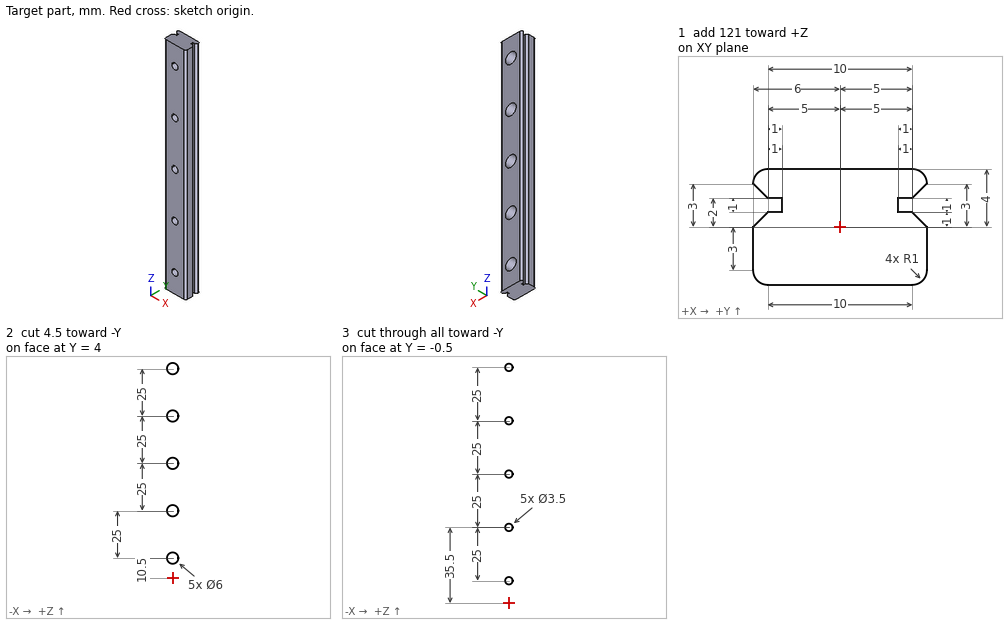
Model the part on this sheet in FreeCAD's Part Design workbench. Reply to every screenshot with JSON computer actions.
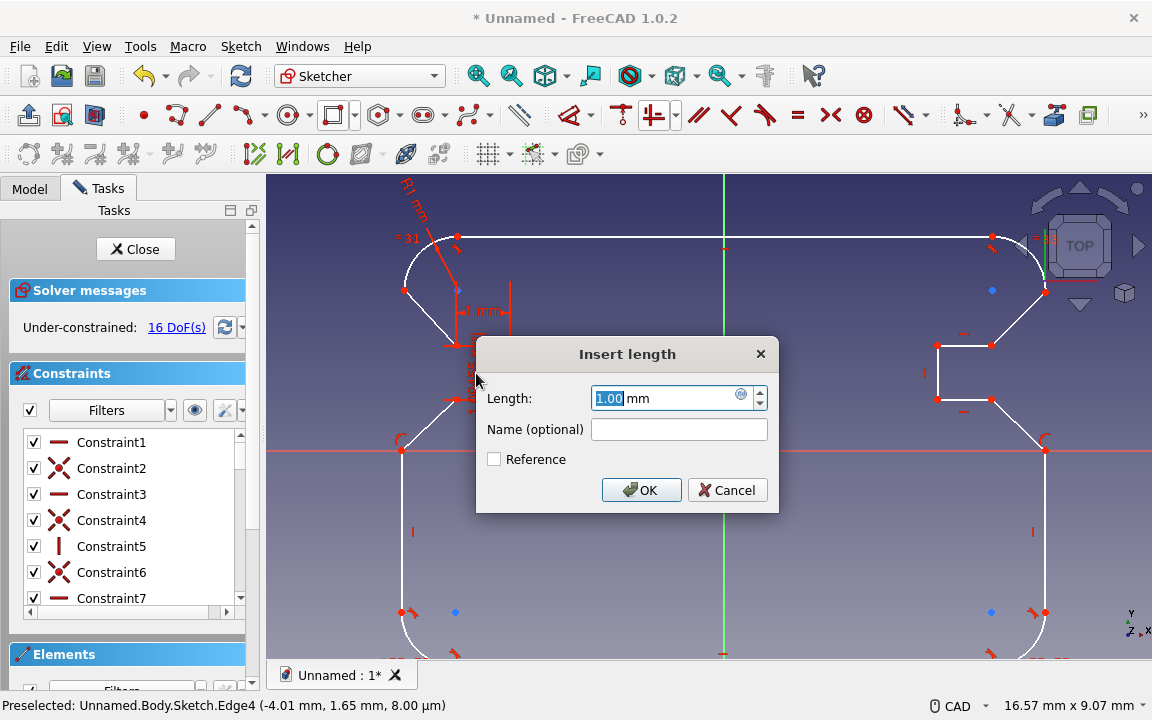
{"action": "type", "text": "1"}
{"action": "key", "text": "Return"}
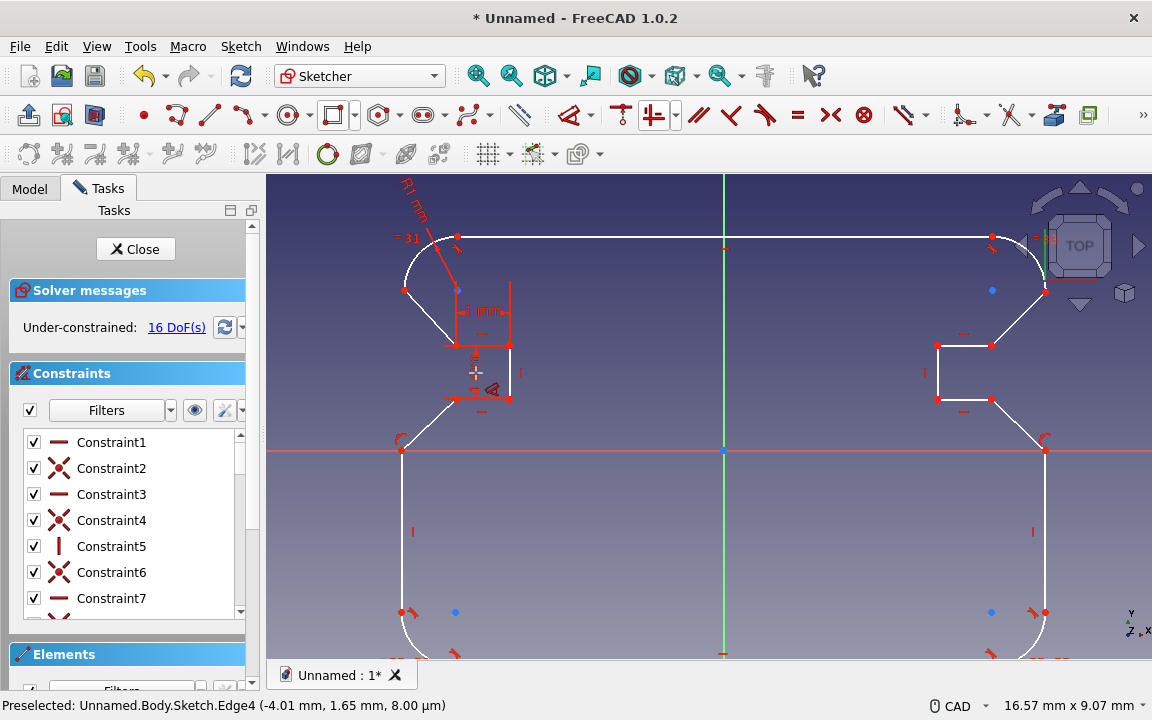
{"action": "left_click", "coordinate": [494, 399]}
{"action": "left_click", "coordinate": [483, 433]}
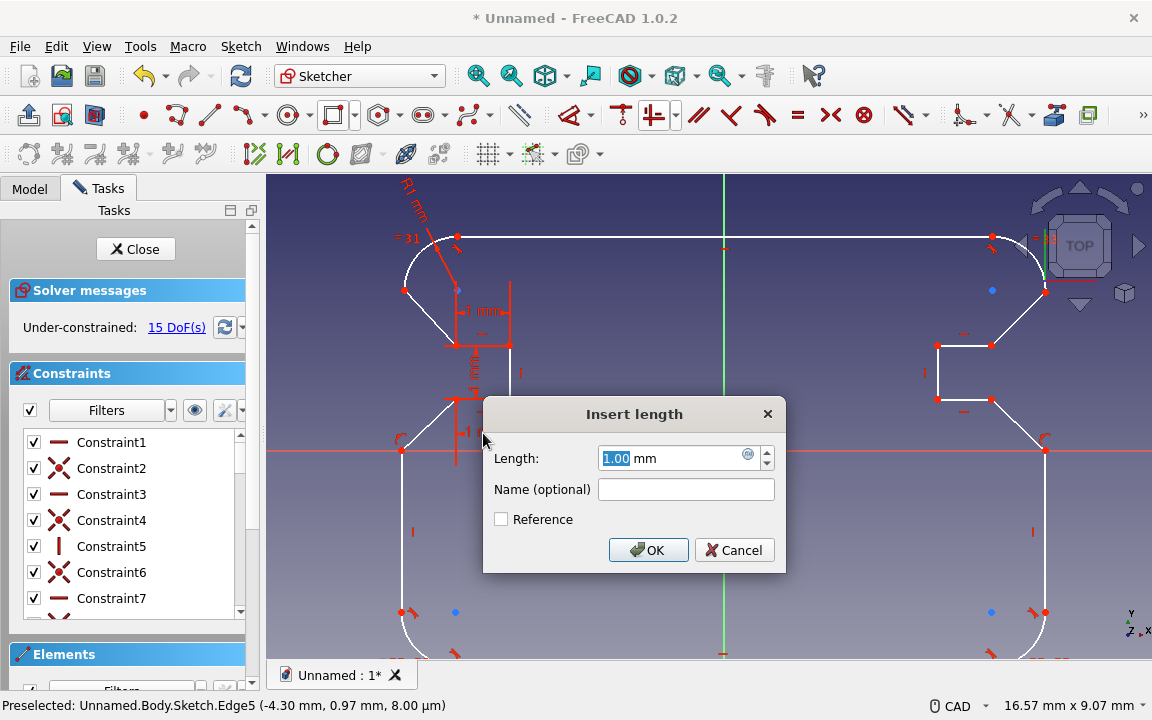
{"action": "type", "text": "1"}
{"action": "key", "text": "Return"}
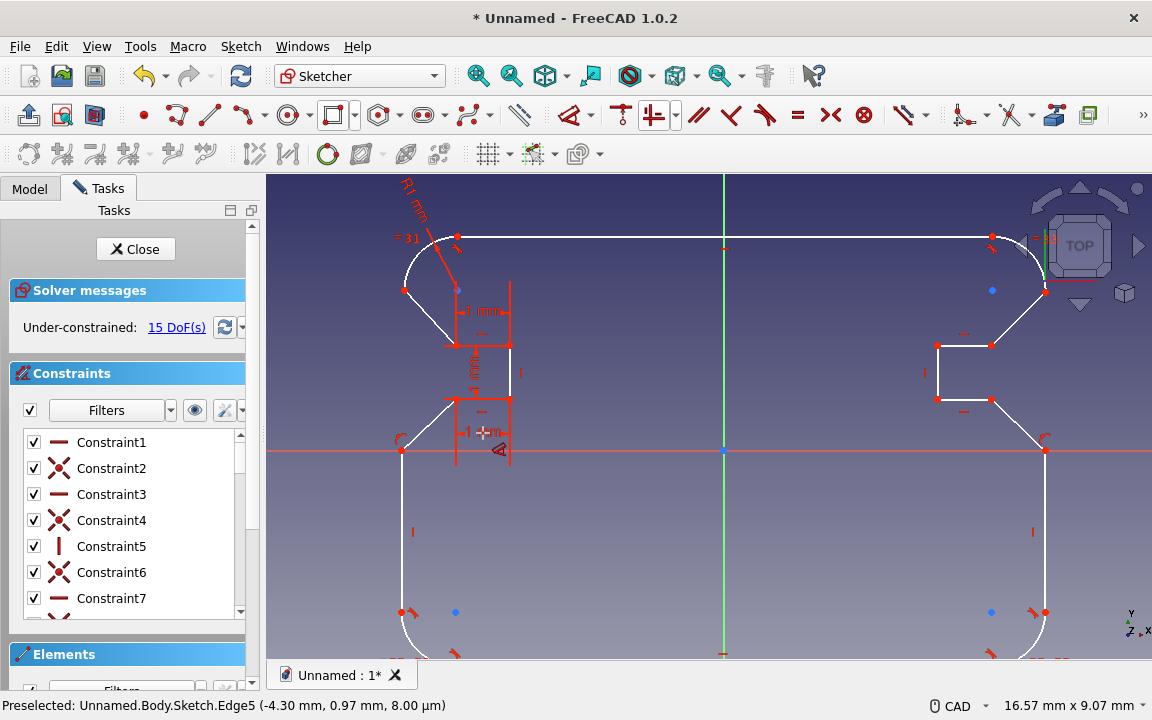
{"action": "left_click", "coordinate": [402, 499]}
{"action": "left_click", "coordinate": [368, 532]}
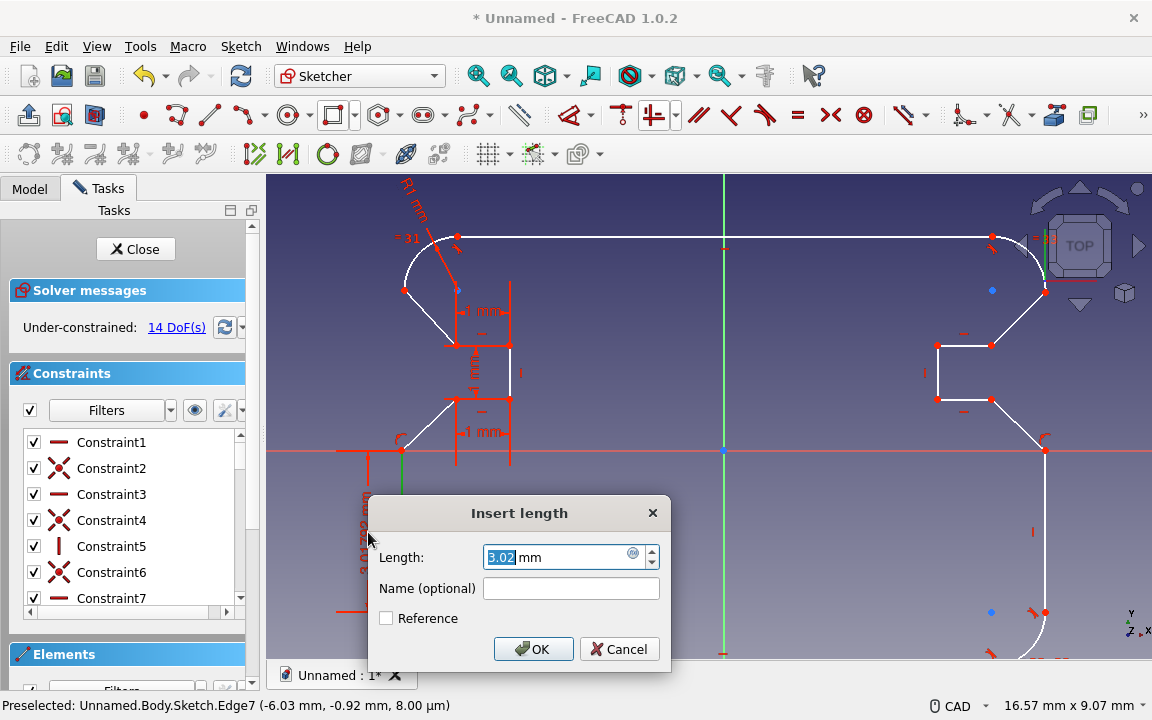
{"action": "type", "text": "3"}
{"action": "key", "text": "Return"}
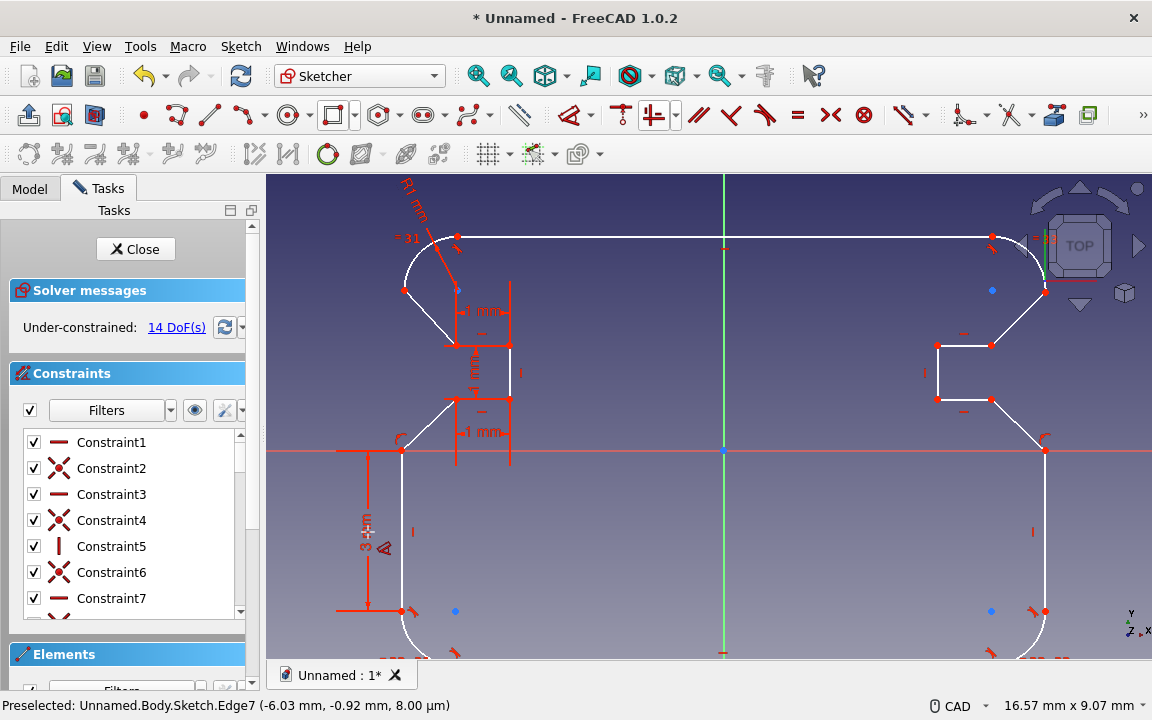
{"action": "left_click", "coordinate": [976, 400]}
{"action": "left_click", "coordinate": [962, 366]}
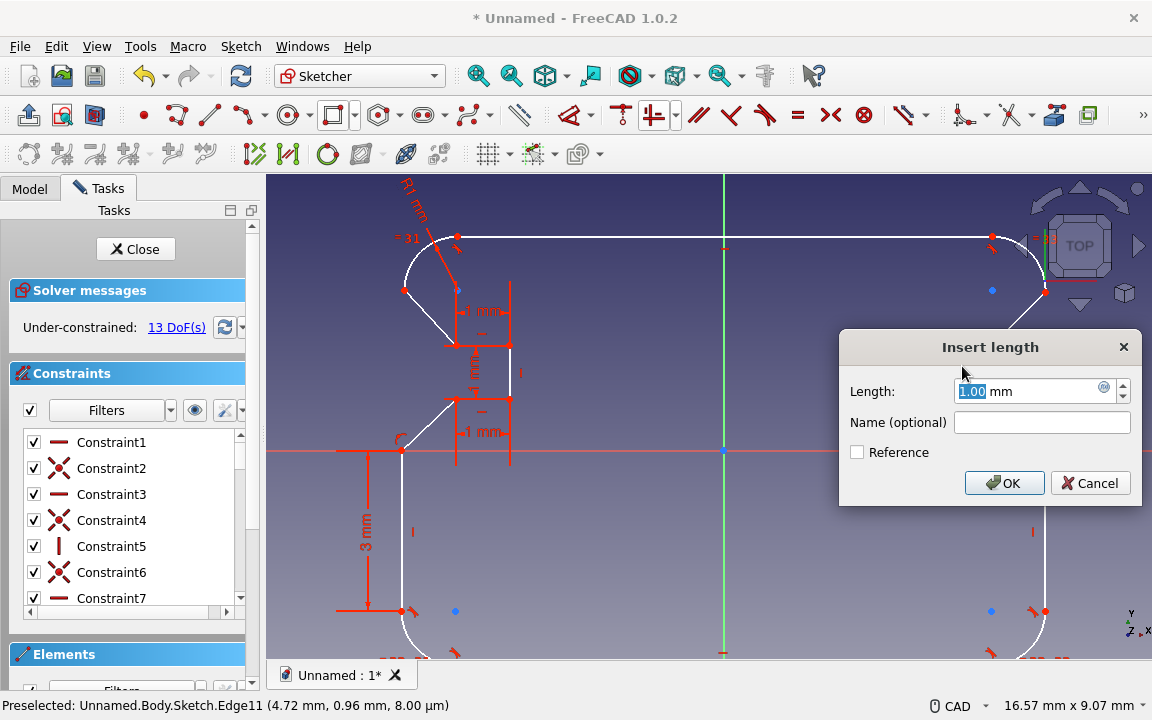
{"action": "type", "text": "1"}
{"action": "key", "text": "Return"}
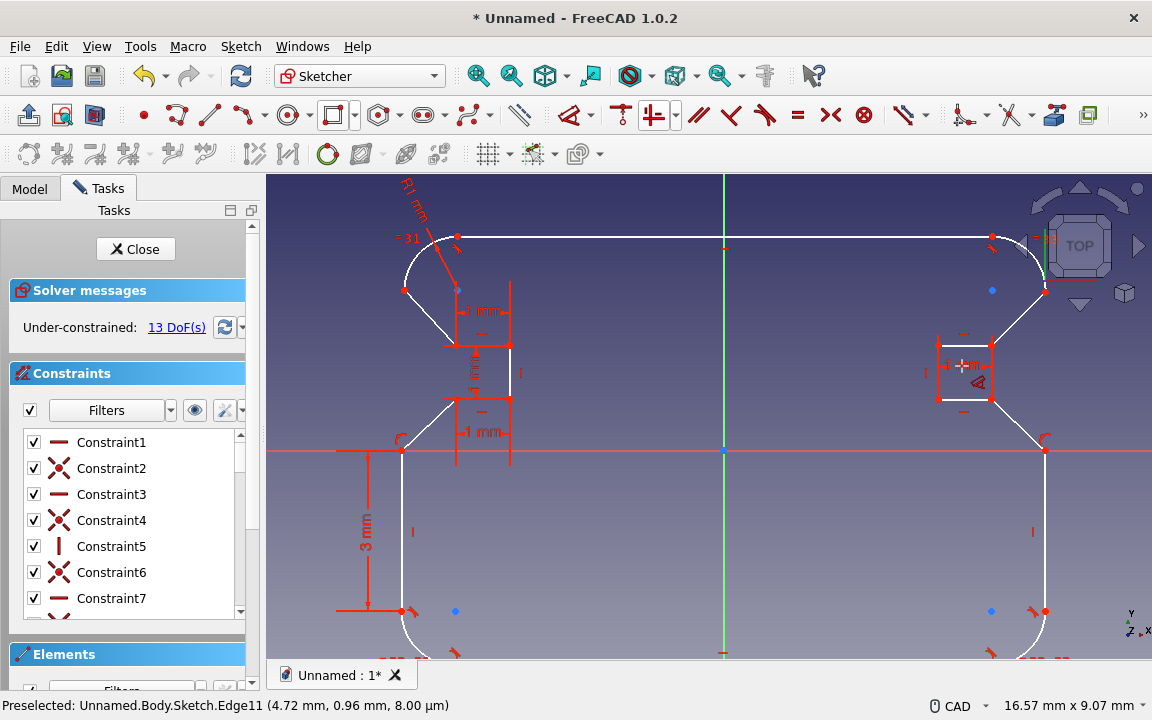
{"action": "left_click", "coordinate": [938, 383]}
{"action": "left_click", "coordinate": [904, 391]}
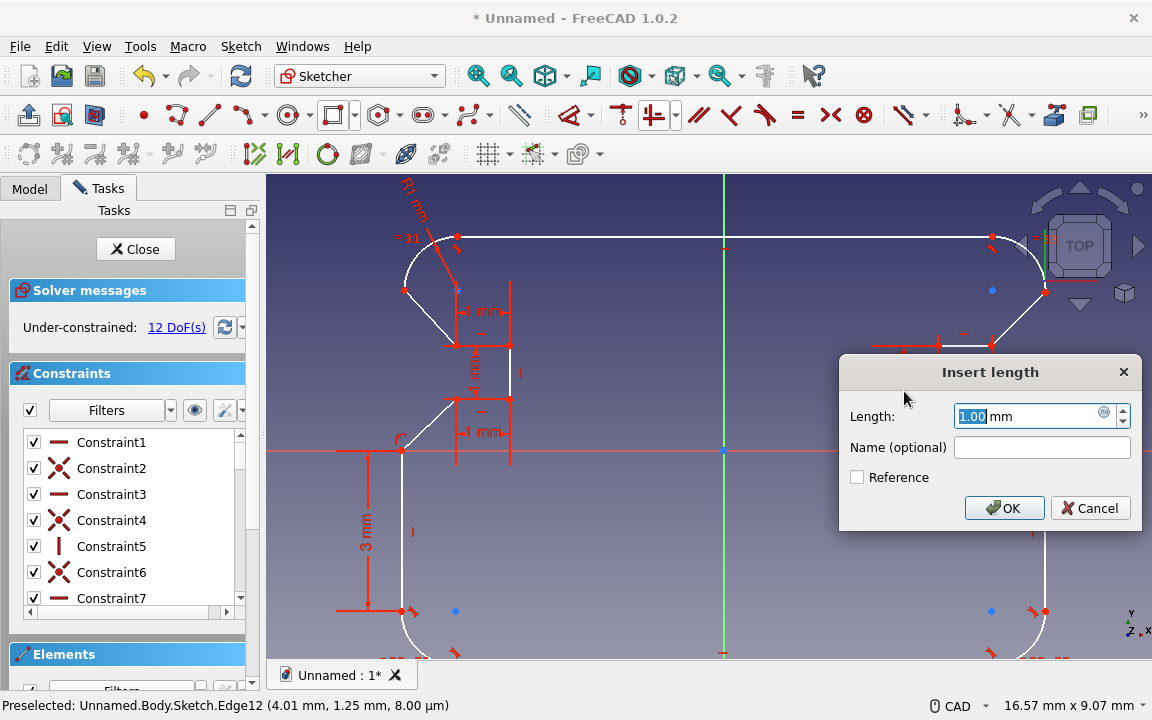
{"action": "type", "text": "1"}
{"action": "key", "text": "Return"}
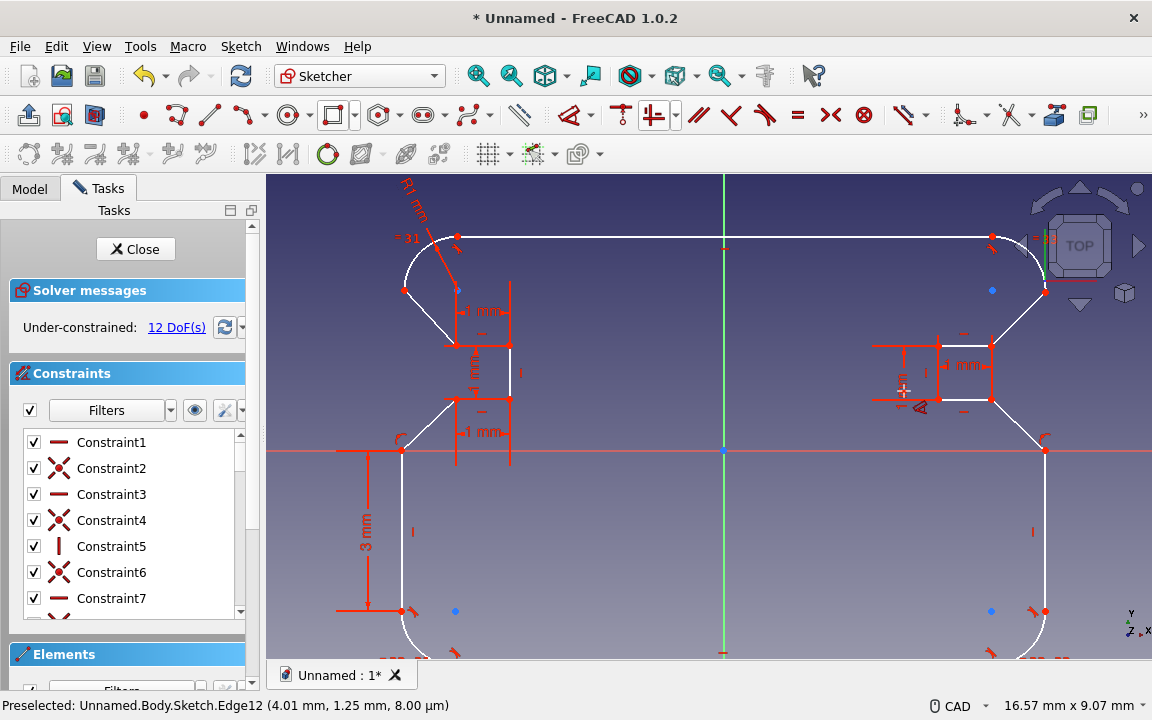
{"action": "left_click", "coordinate": [954, 346]}
{"action": "left_click", "coordinate": [963, 312]}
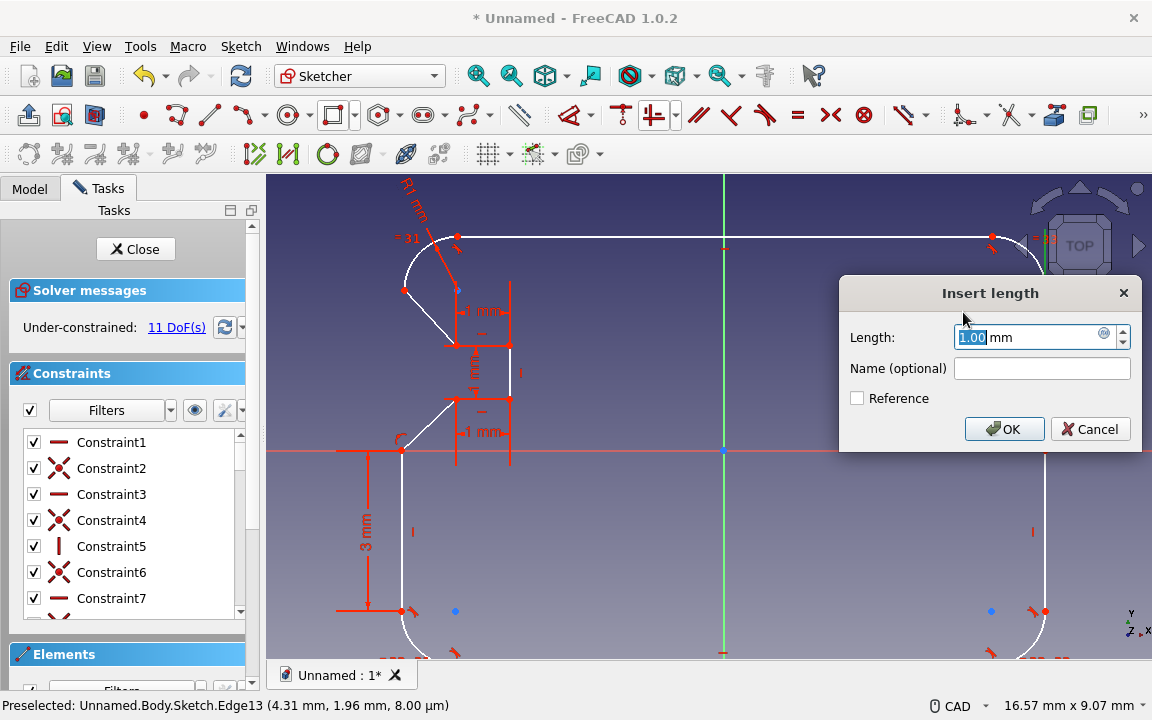
{"action": "type", "text": "1"}
{"action": "key", "text": "Return"}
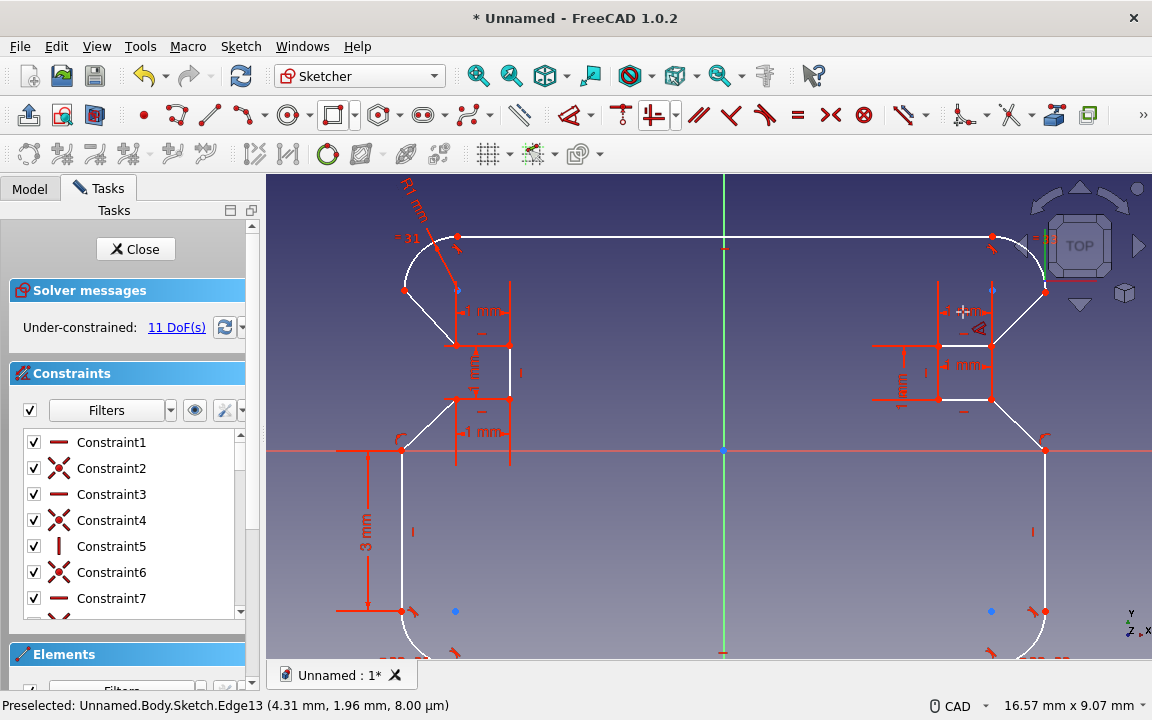
{"action": "left_click", "coordinate": [832, 237]}
{"action": "left_click", "coordinate": [601, 203]}